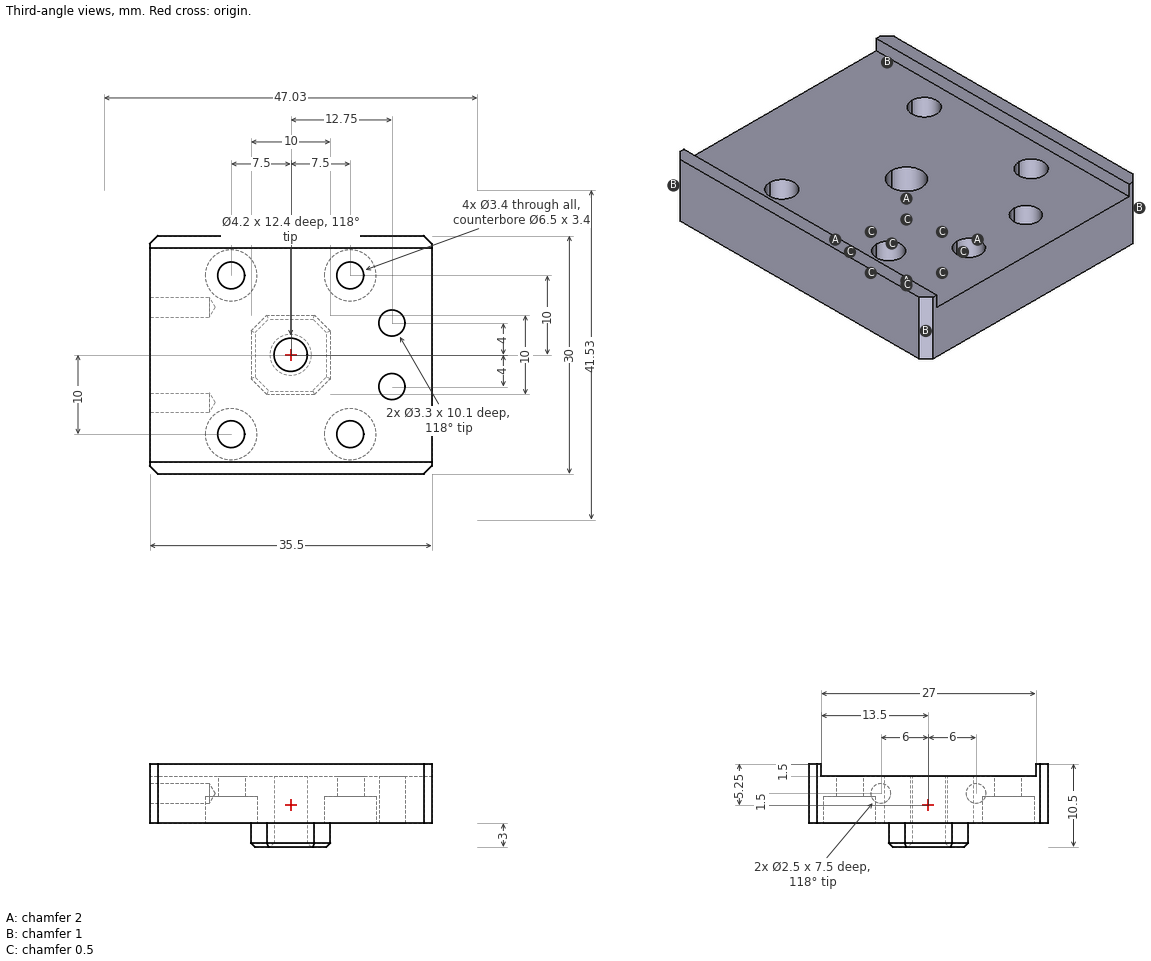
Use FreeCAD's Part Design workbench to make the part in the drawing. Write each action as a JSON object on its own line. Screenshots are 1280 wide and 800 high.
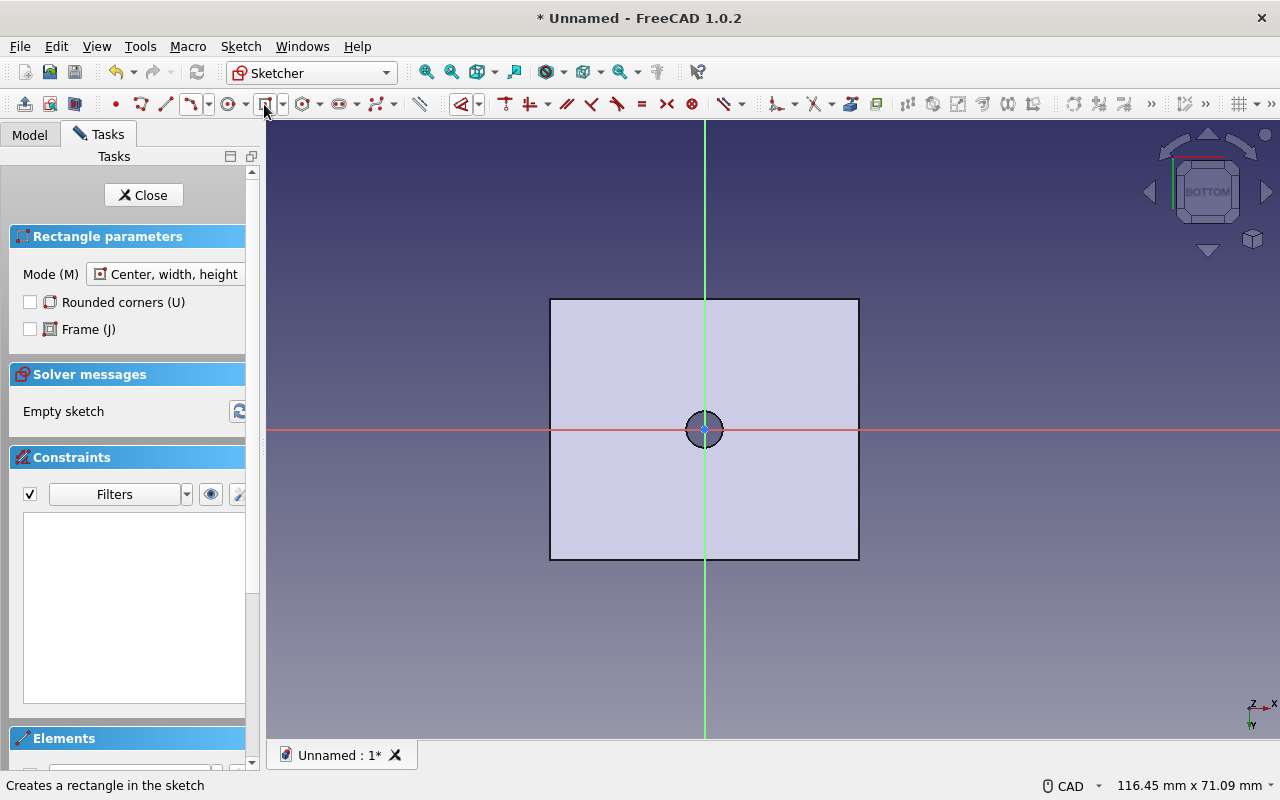
{"action": "left_click", "coordinate": [705, 430]}
{"action": "left_click", "coordinate": [909, 249]}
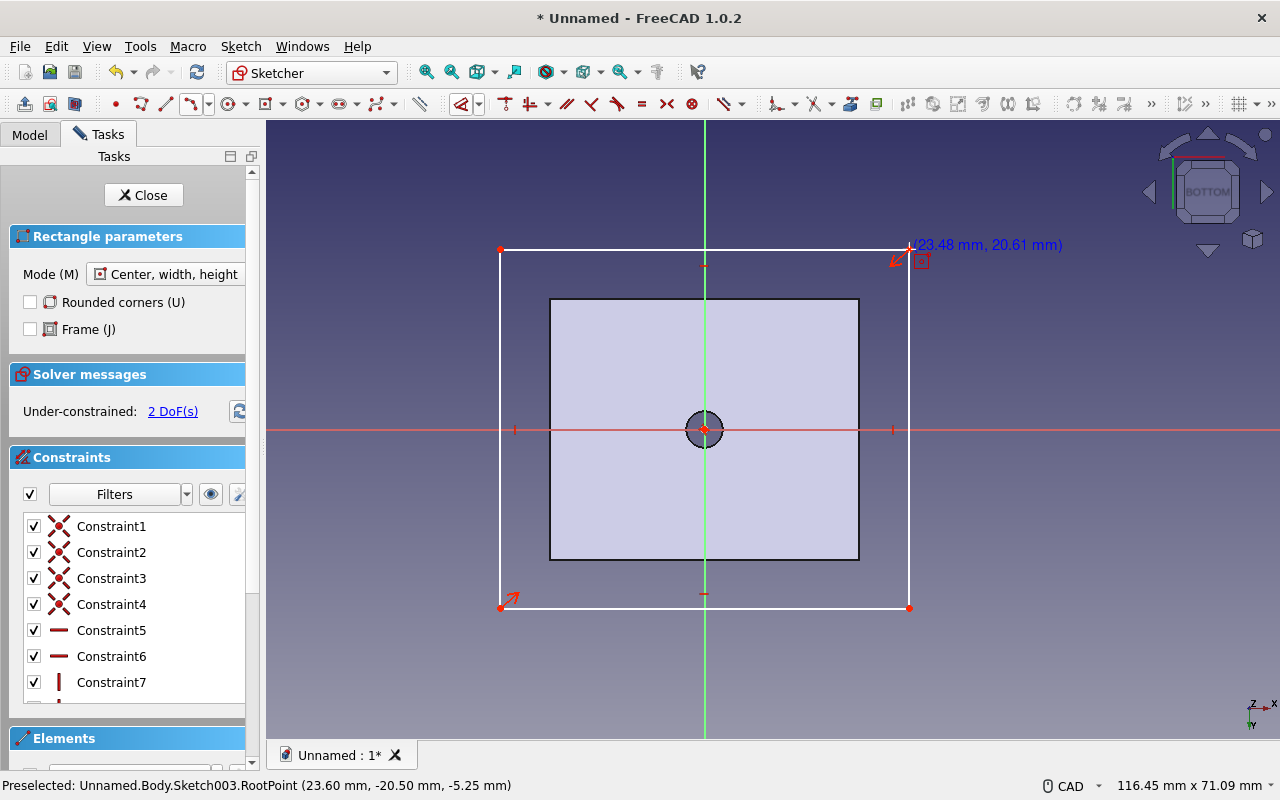
{"action": "left_click", "coordinate": [705, 430]}
{"action": "left_click", "coordinate": [748, 386]}
{"action": "key", "text": "Escape"}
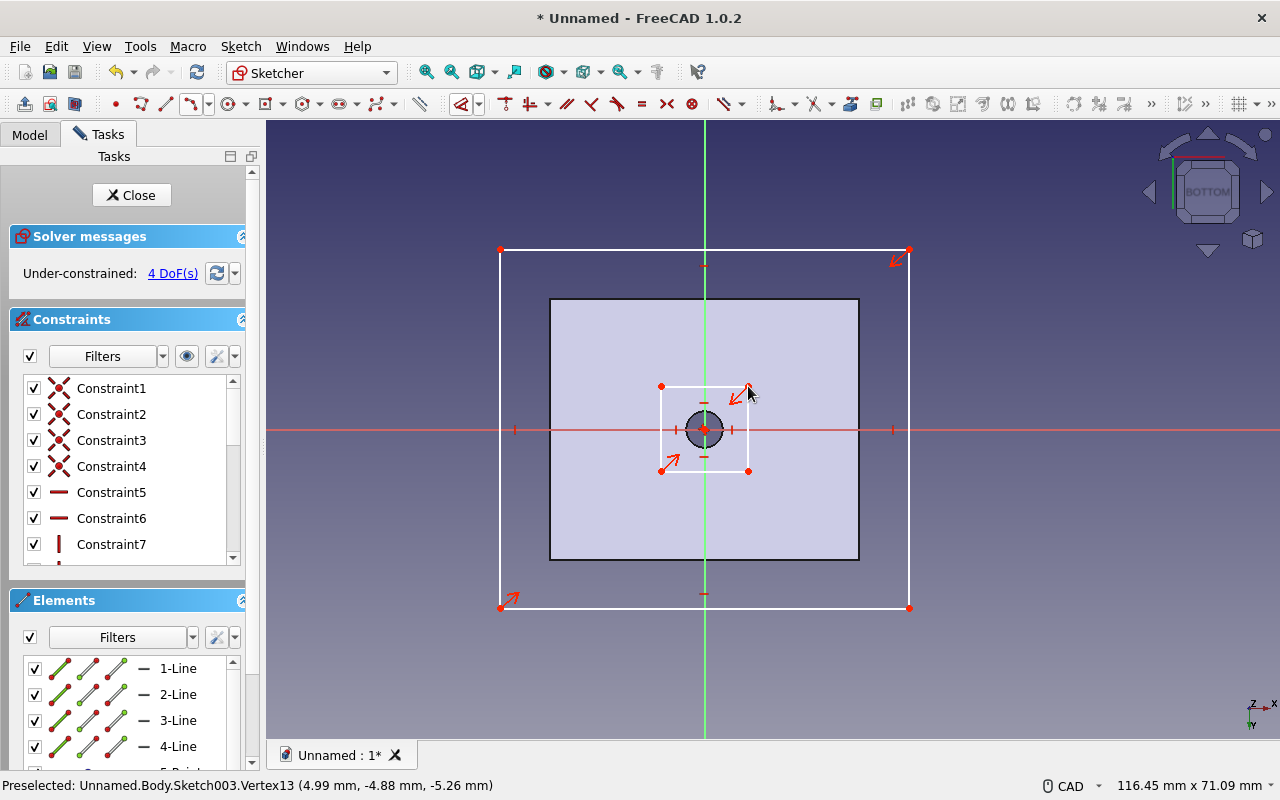
{"action": "key", "text": "d"}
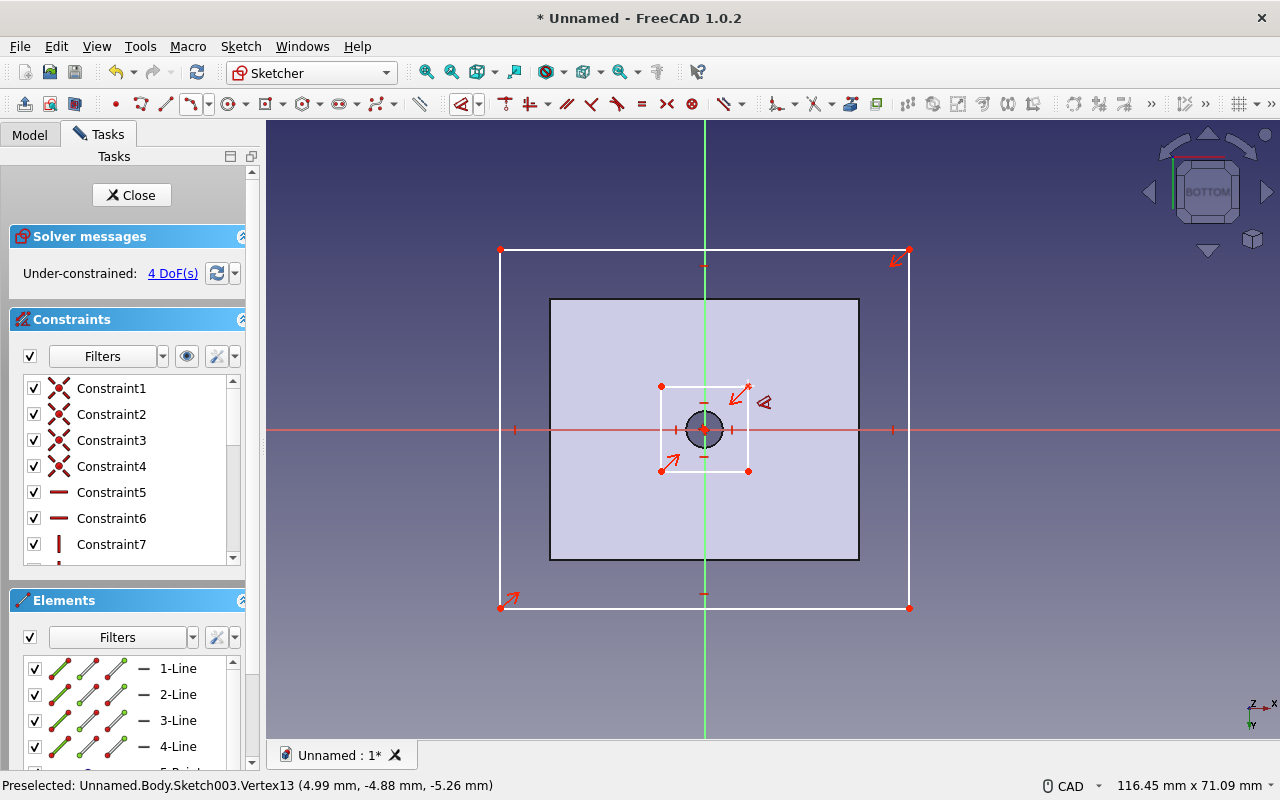
{"action": "left_click", "coordinate": [687, 472]}
{"action": "left_click", "coordinate": [685, 506]}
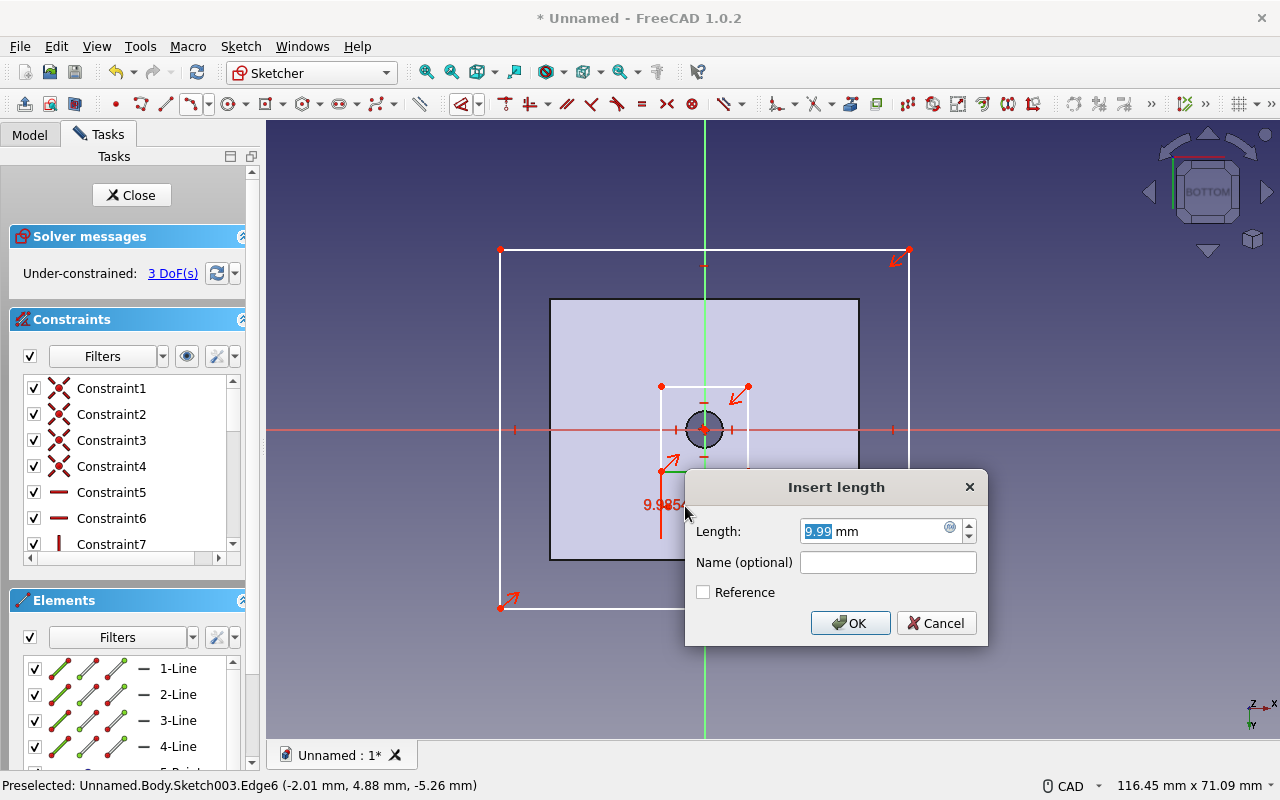
{"action": "type", "text": "10"}
{"action": "key", "text": "Return"}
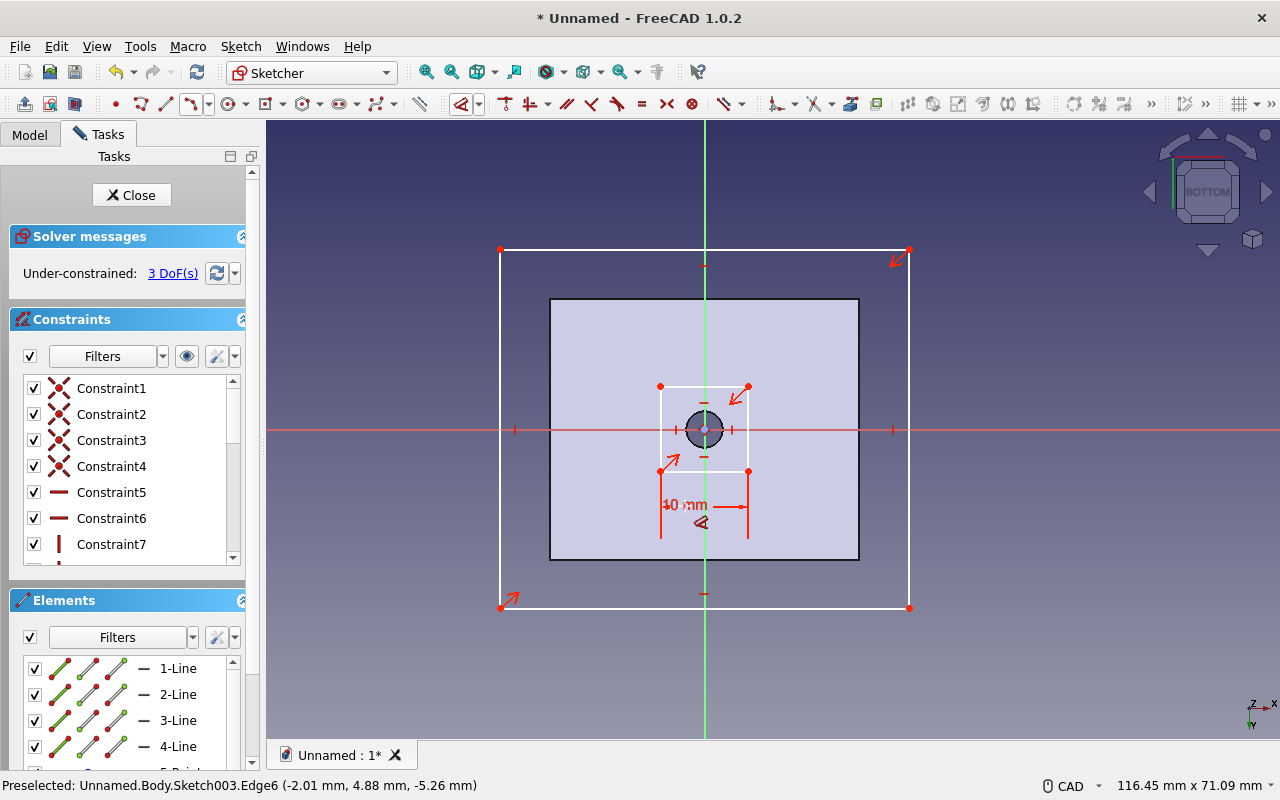
{"action": "left_click", "coordinate": [748, 447]}
{"action": "left_click", "coordinate": [782, 410]}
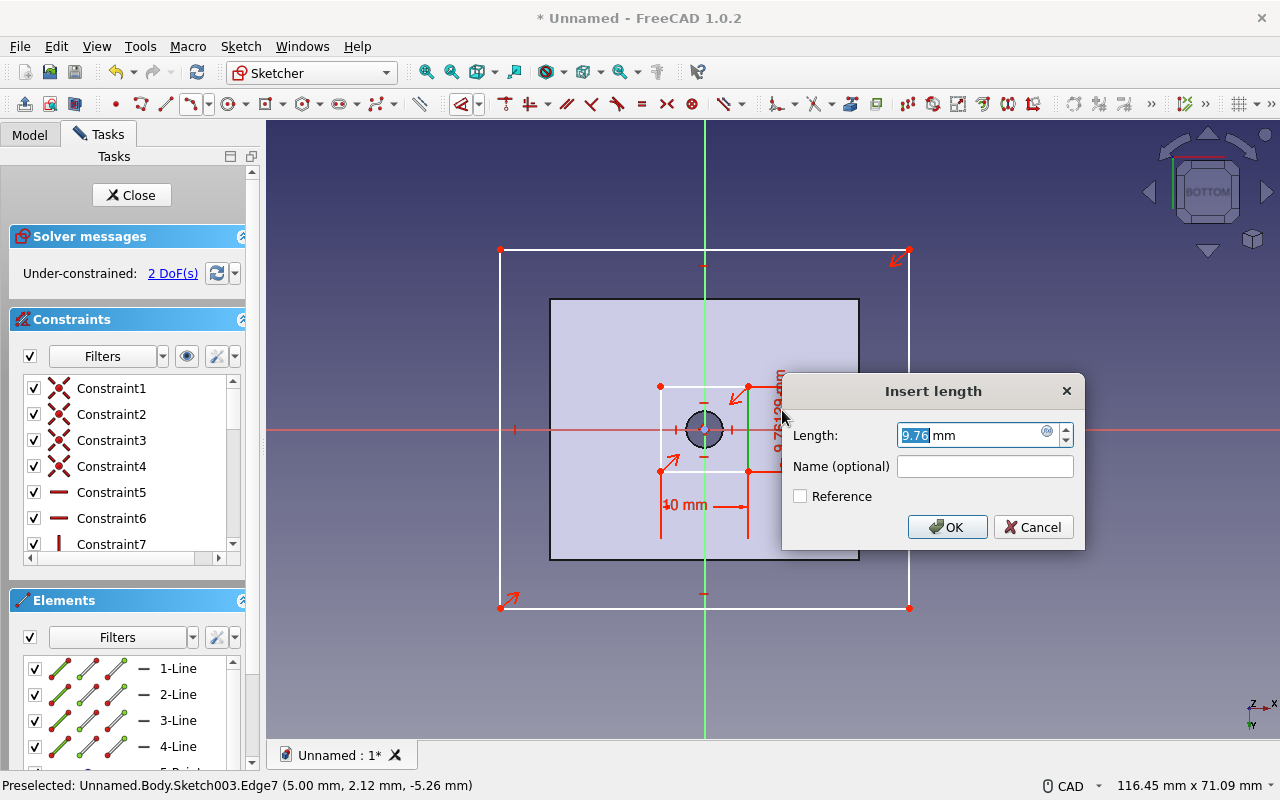
{"action": "type", "text": "10"}
{"action": "key", "text": "Return"}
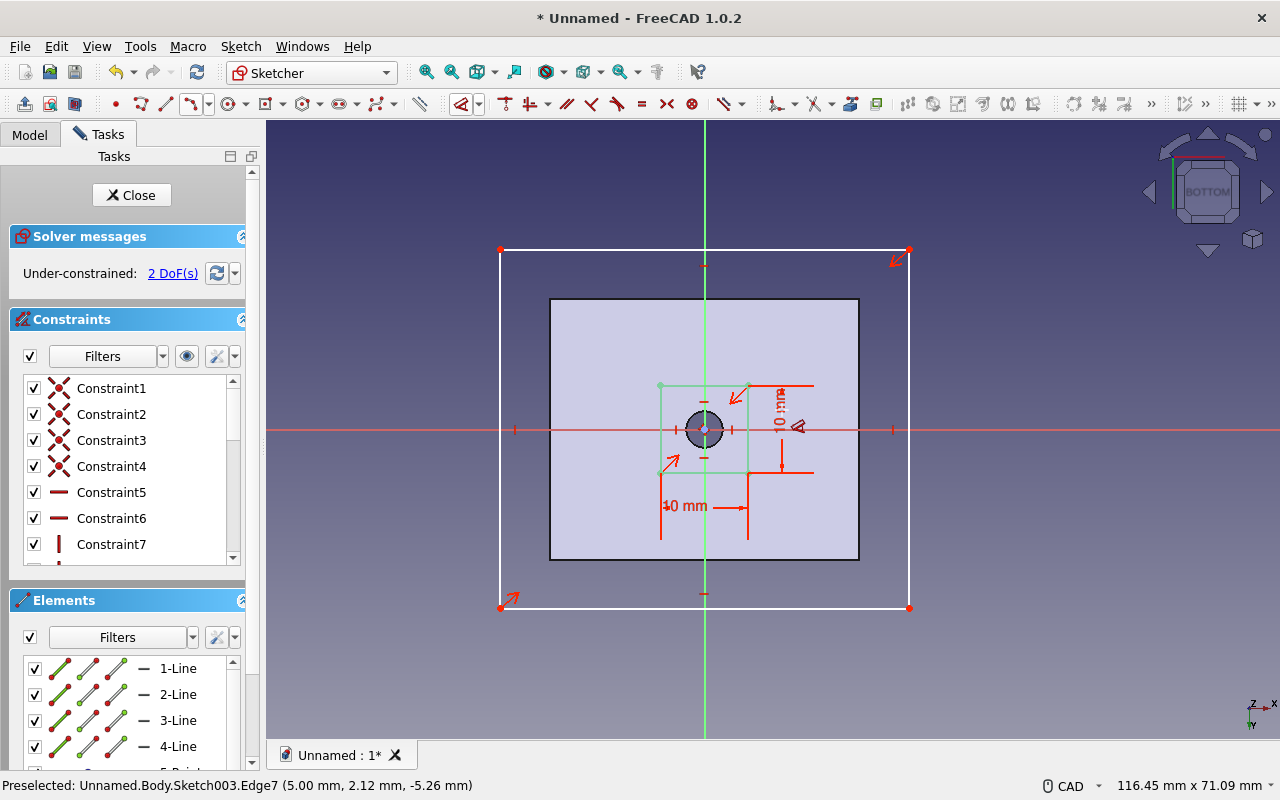
{"action": "left_click", "coordinate": [623, 609]}
{"action": "left_click", "coordinate": [610, 643]}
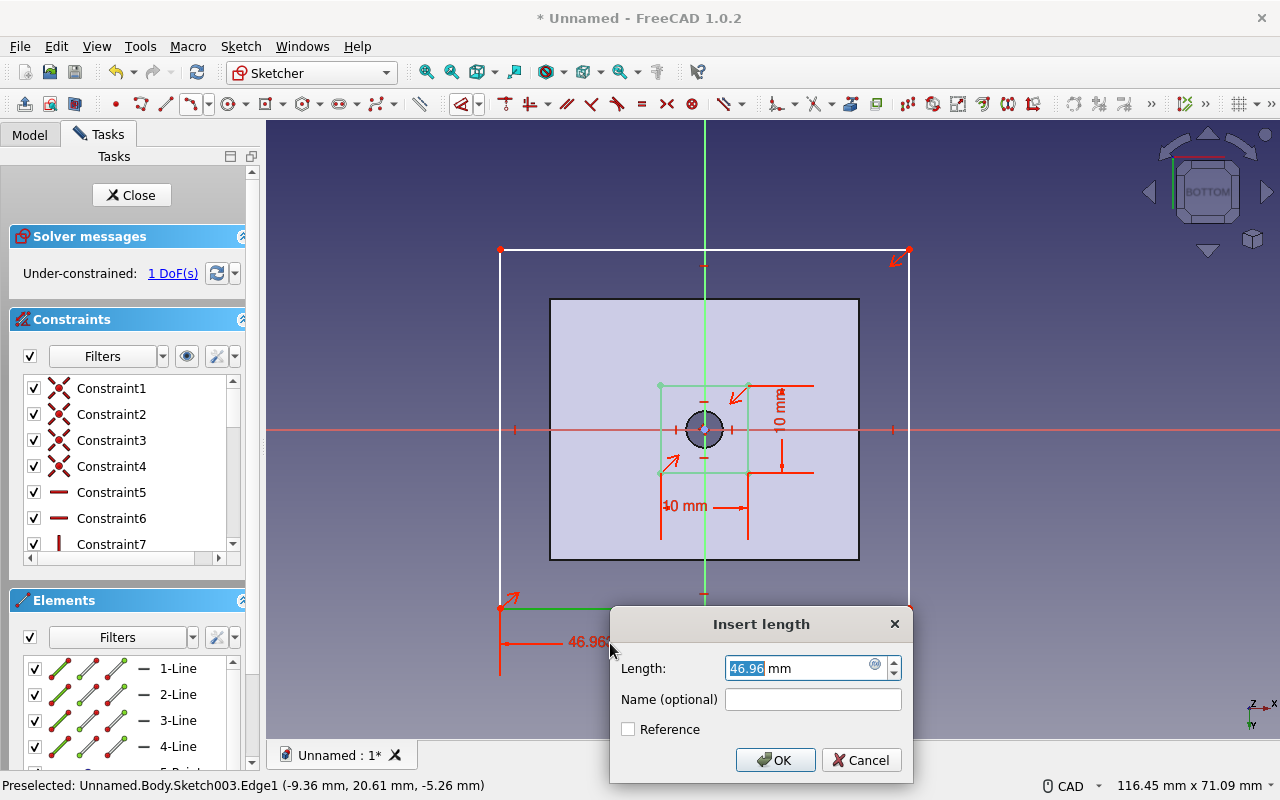
{"action": "type", "text": "47.03"}
{"action": "key", "text": "Return"}